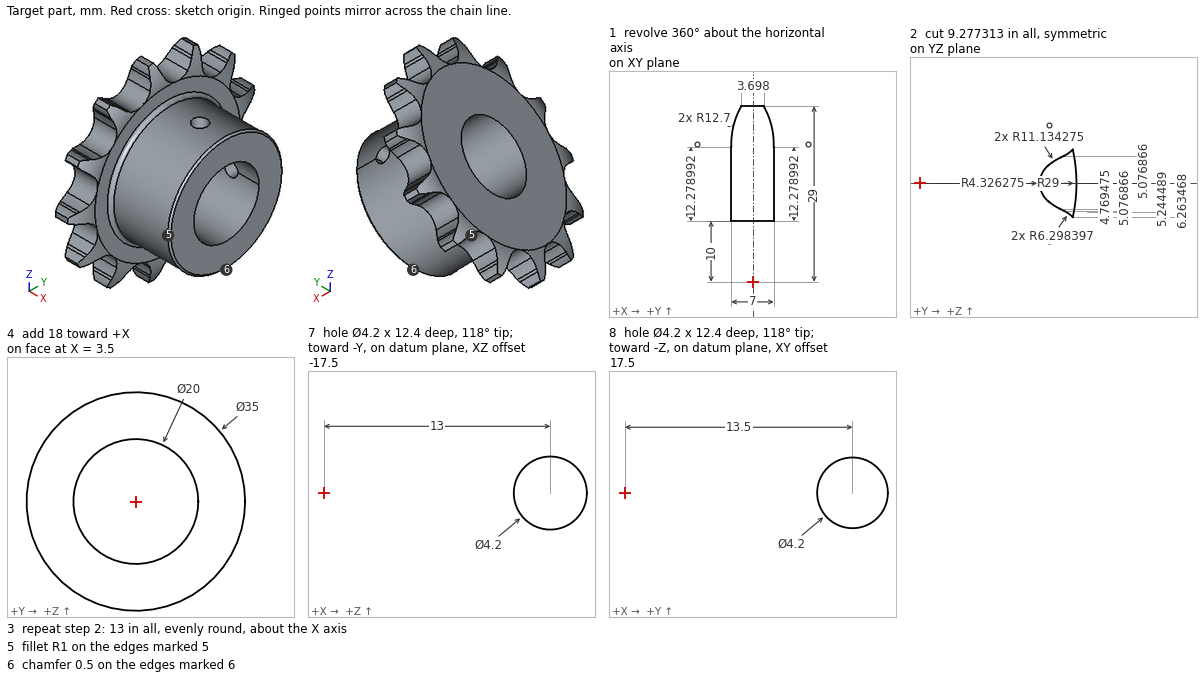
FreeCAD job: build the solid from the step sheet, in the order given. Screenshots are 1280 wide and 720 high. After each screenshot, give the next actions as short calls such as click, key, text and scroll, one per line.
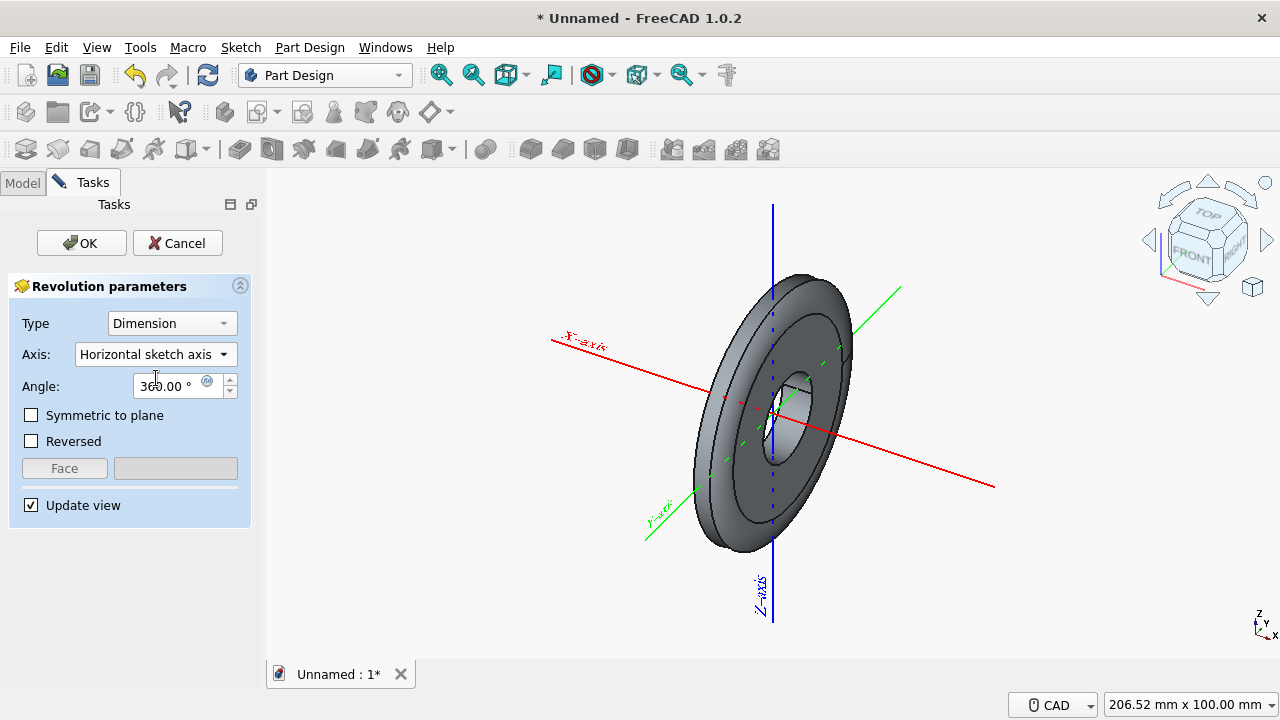
click(82, 243)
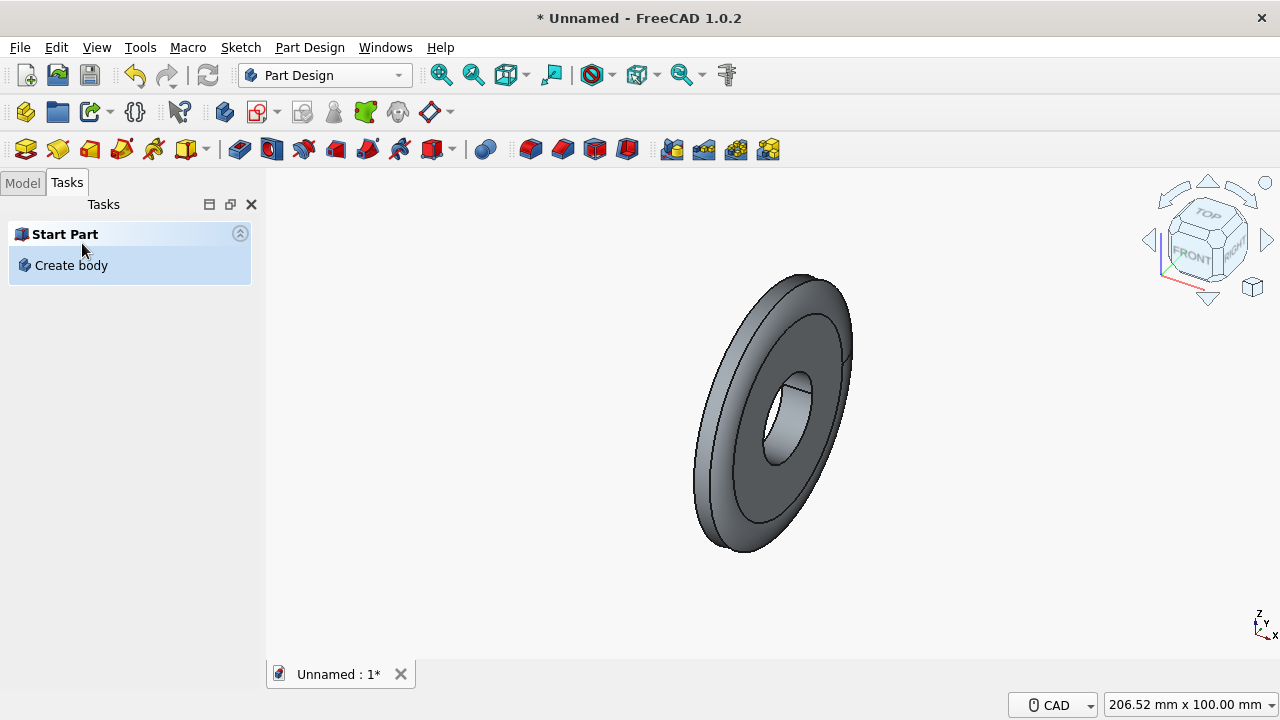
click(258, 112)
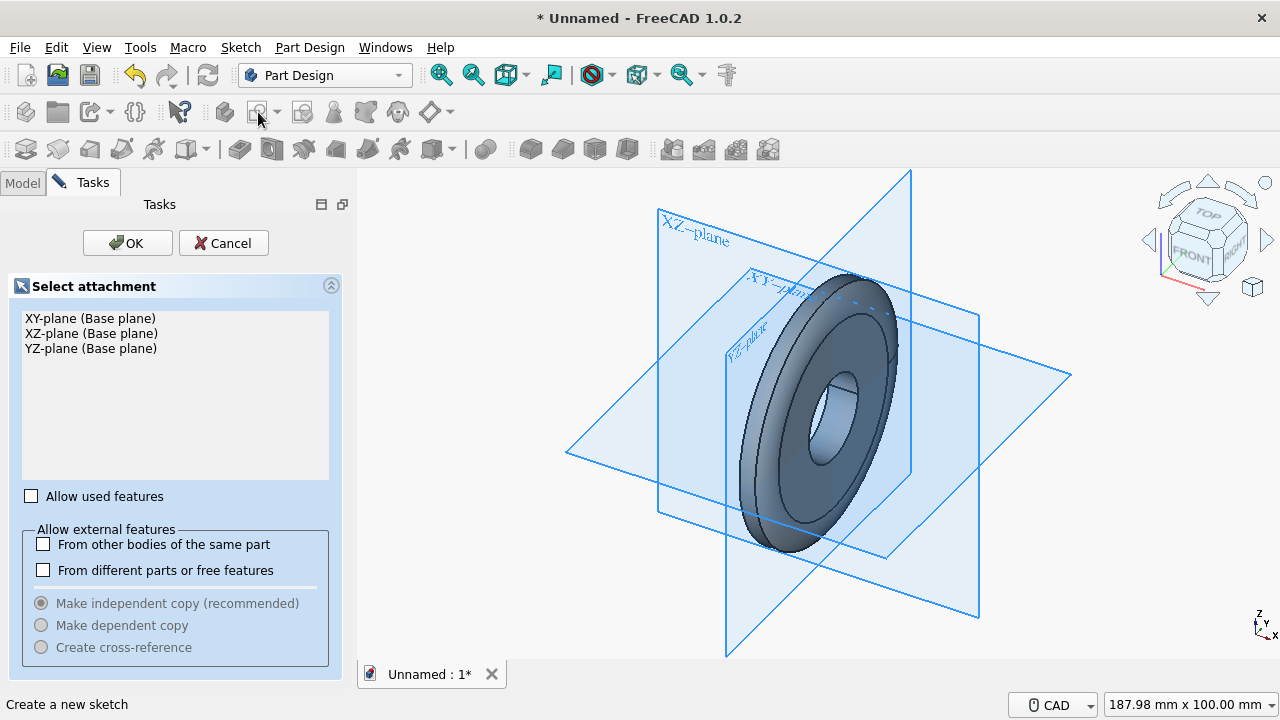
click(82, 348)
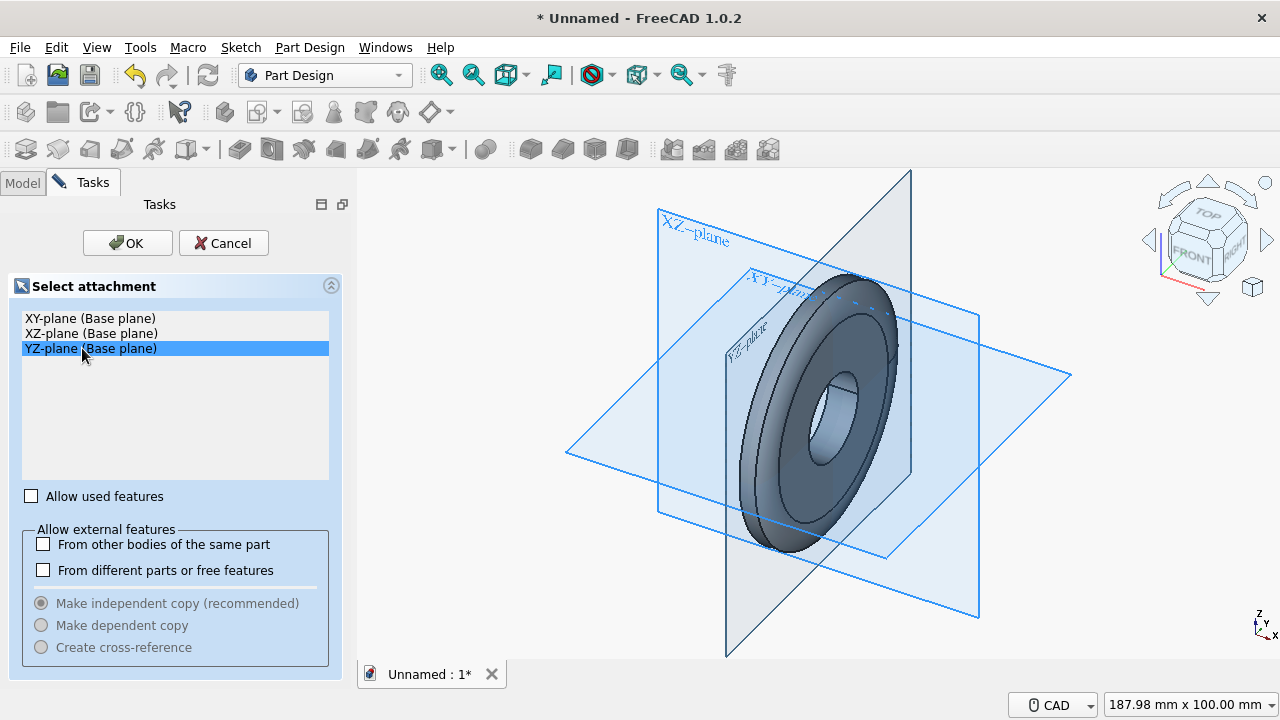
click(128, 243)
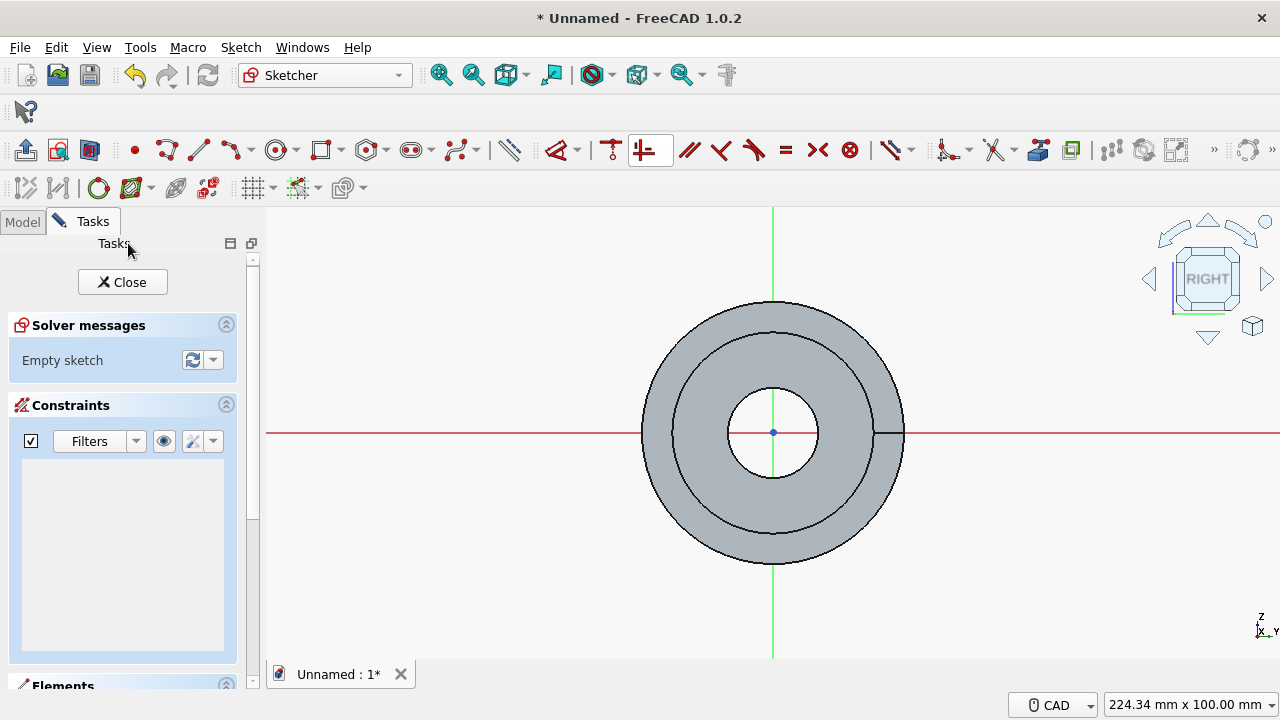
key(q)
key(s)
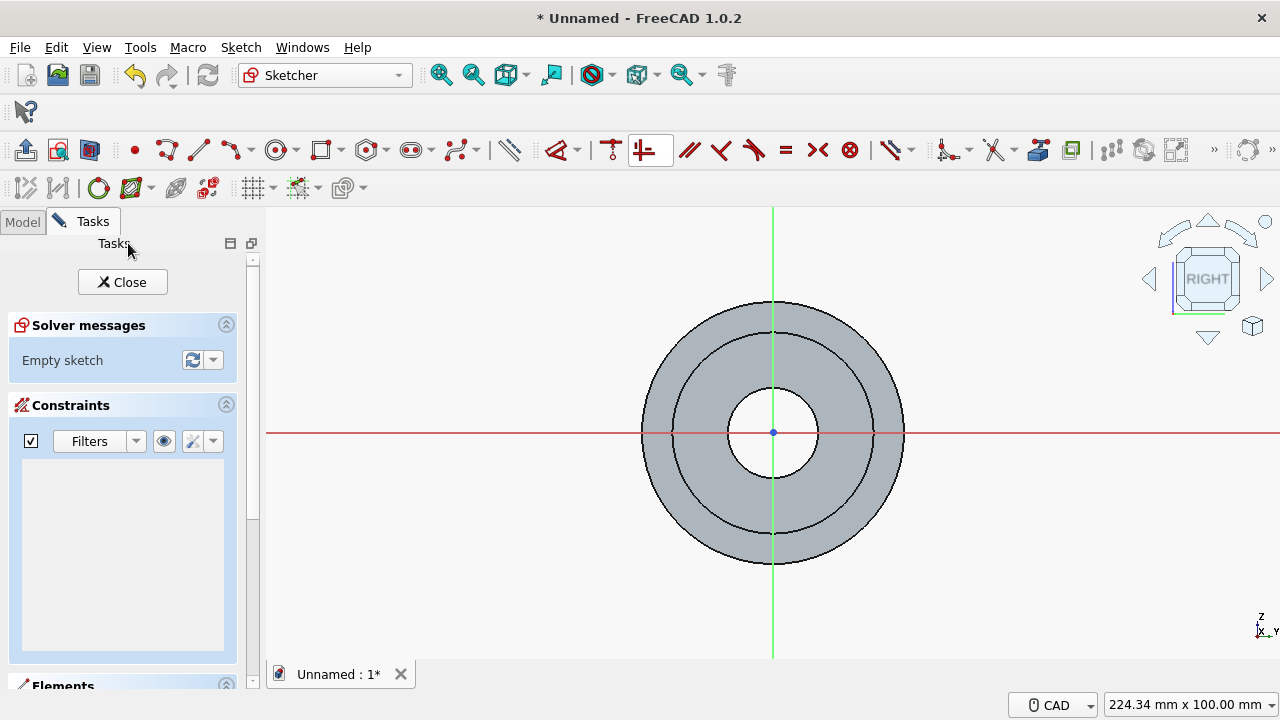
scroll(882, 433, up, 7)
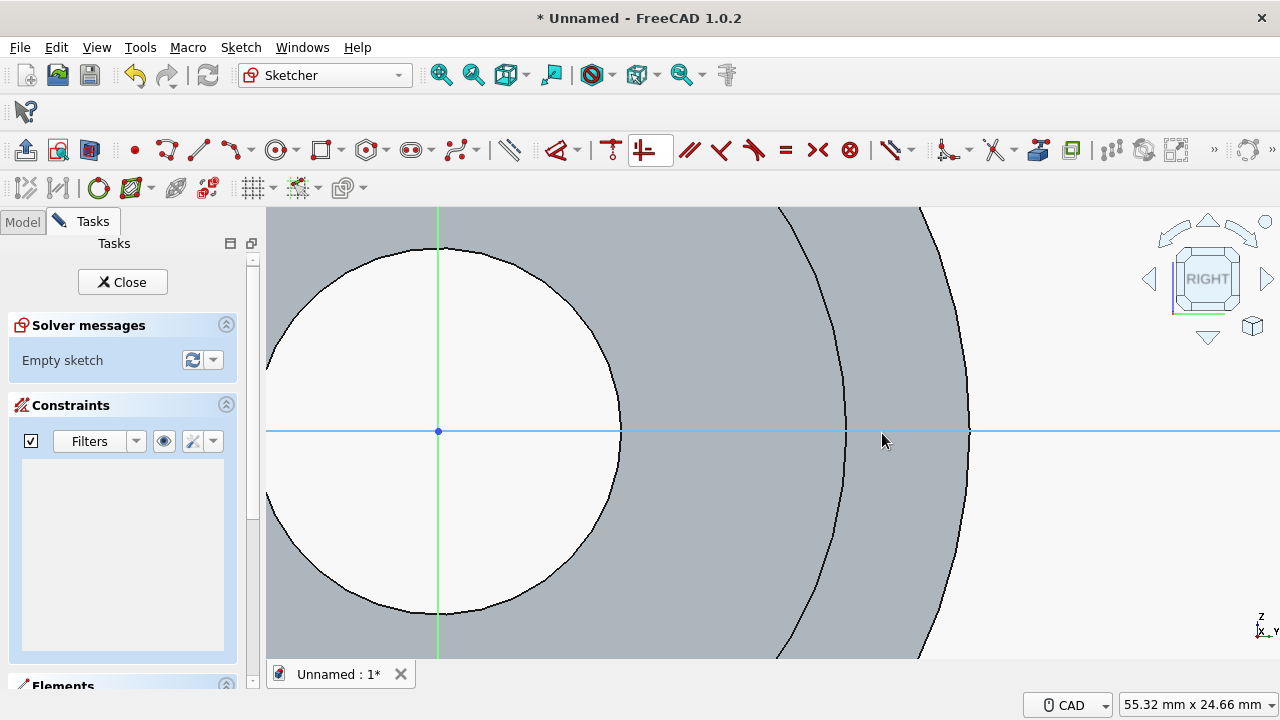
click(200, 150)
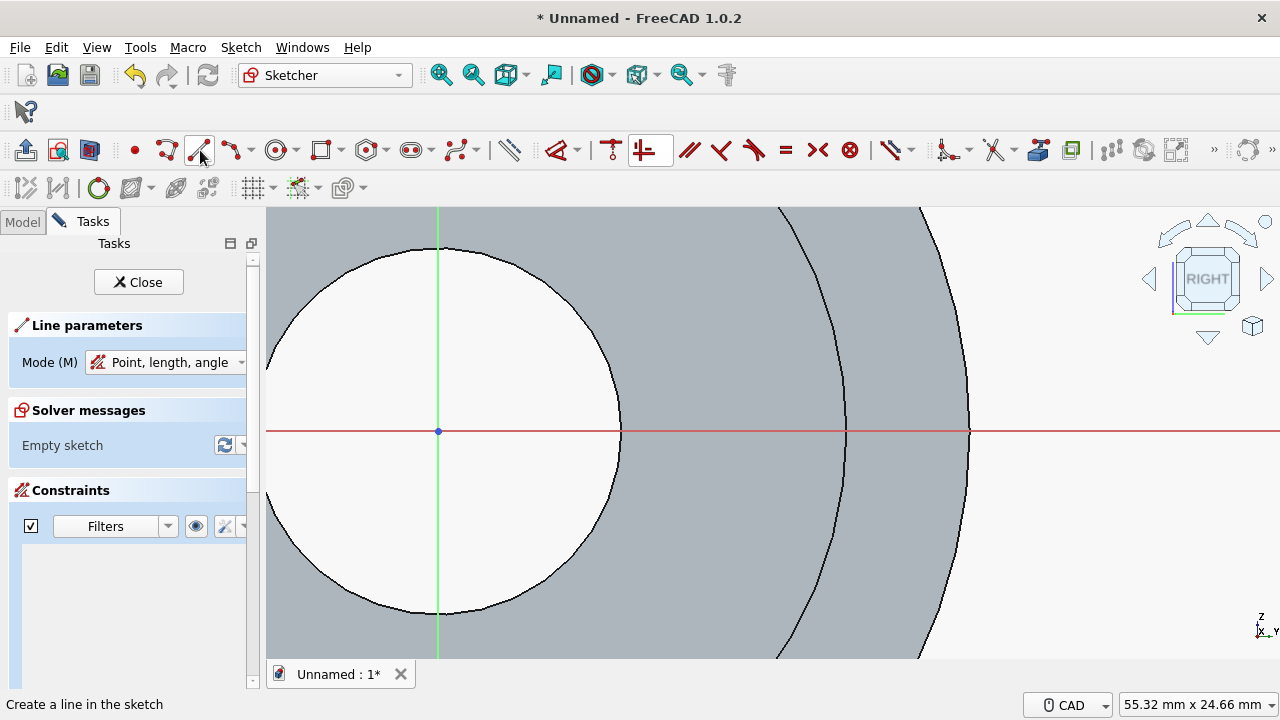
click(915, 519)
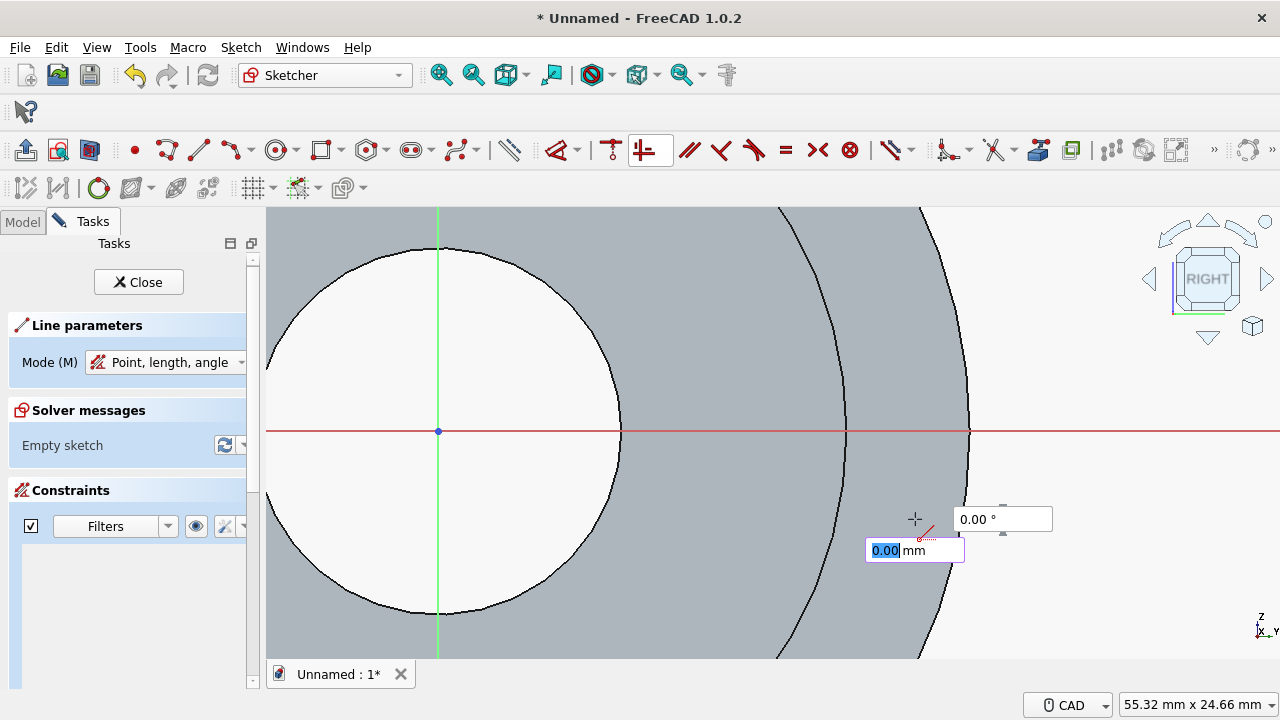
scroll(926, 525, up, 2)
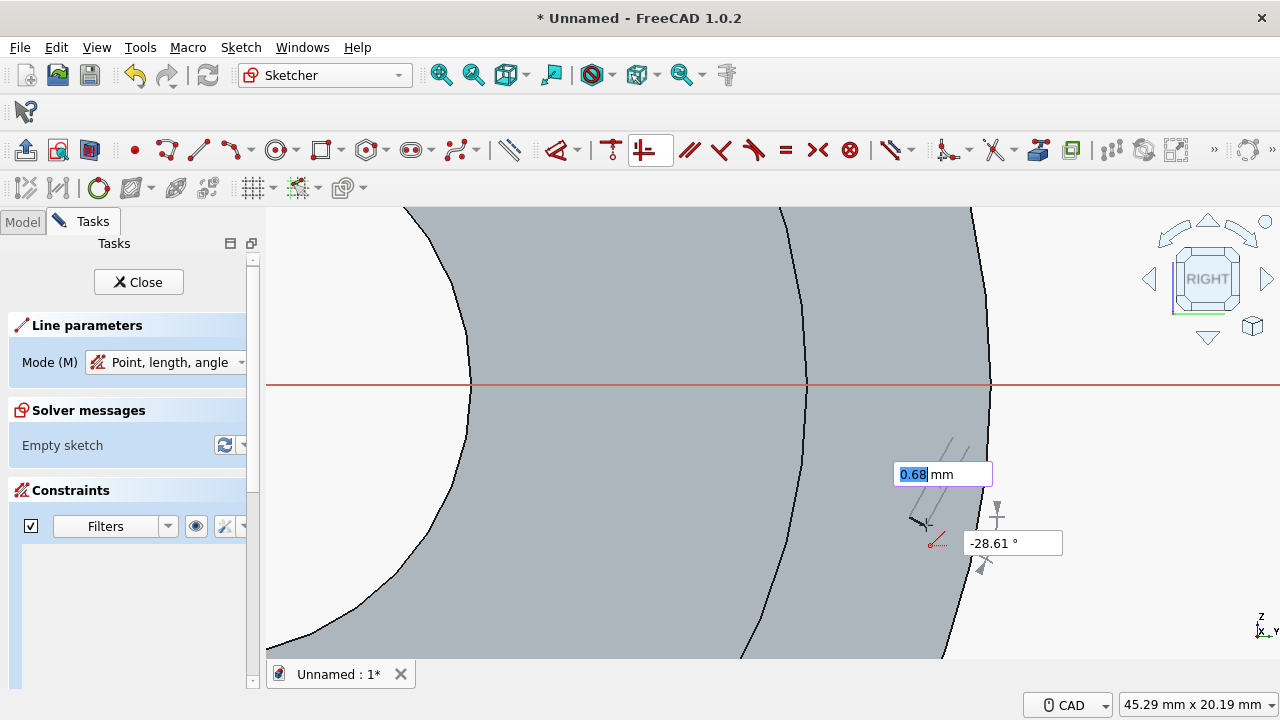
click(926, 524)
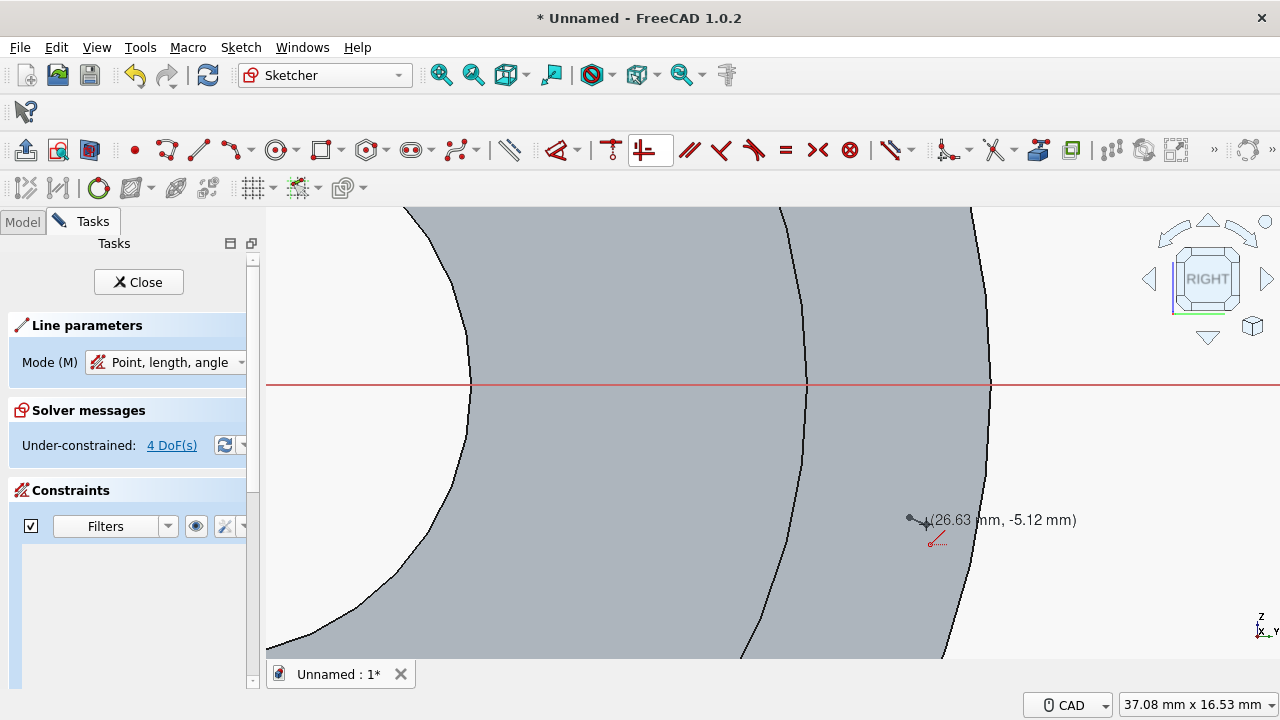
click(926, 246)
click(909, 255)